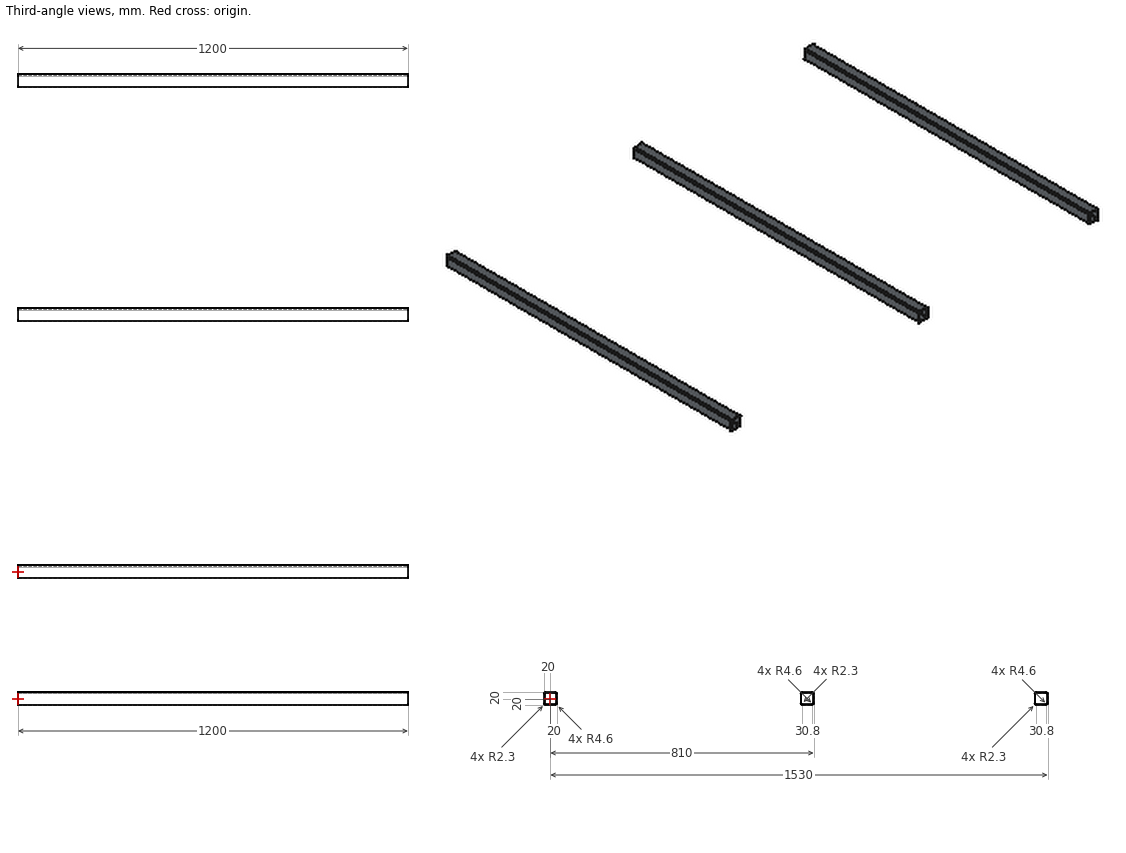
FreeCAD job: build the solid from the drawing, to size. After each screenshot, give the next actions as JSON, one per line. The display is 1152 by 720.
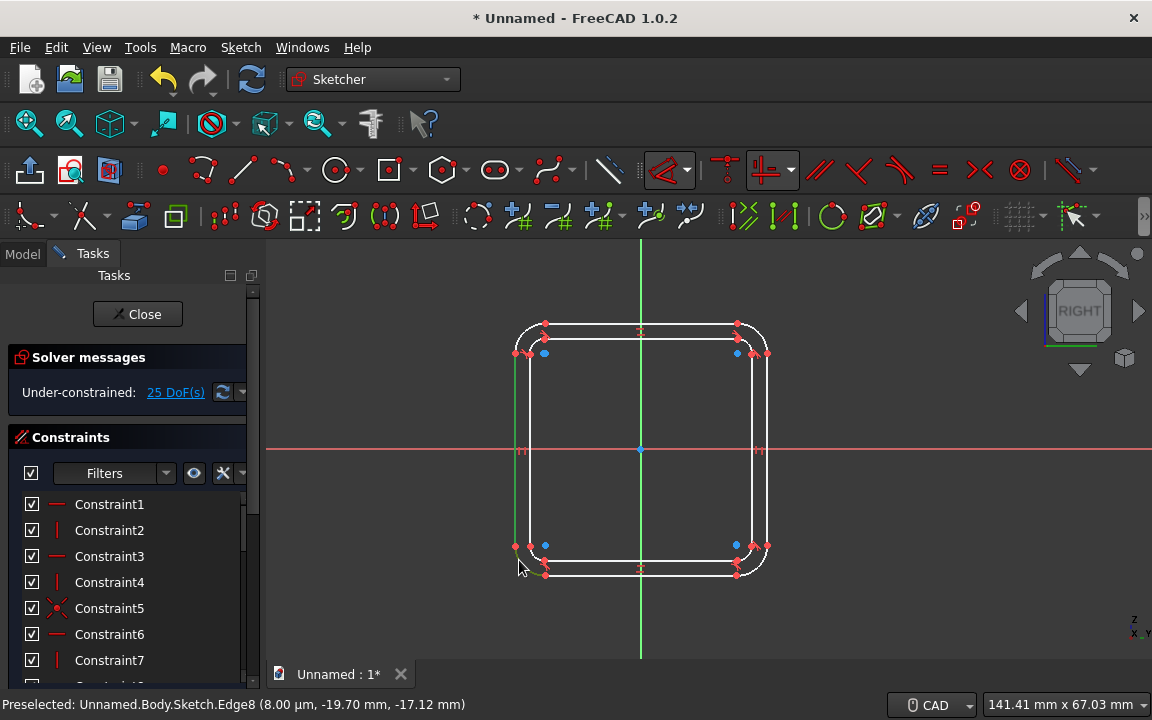
{"action": "key", "text": "t"}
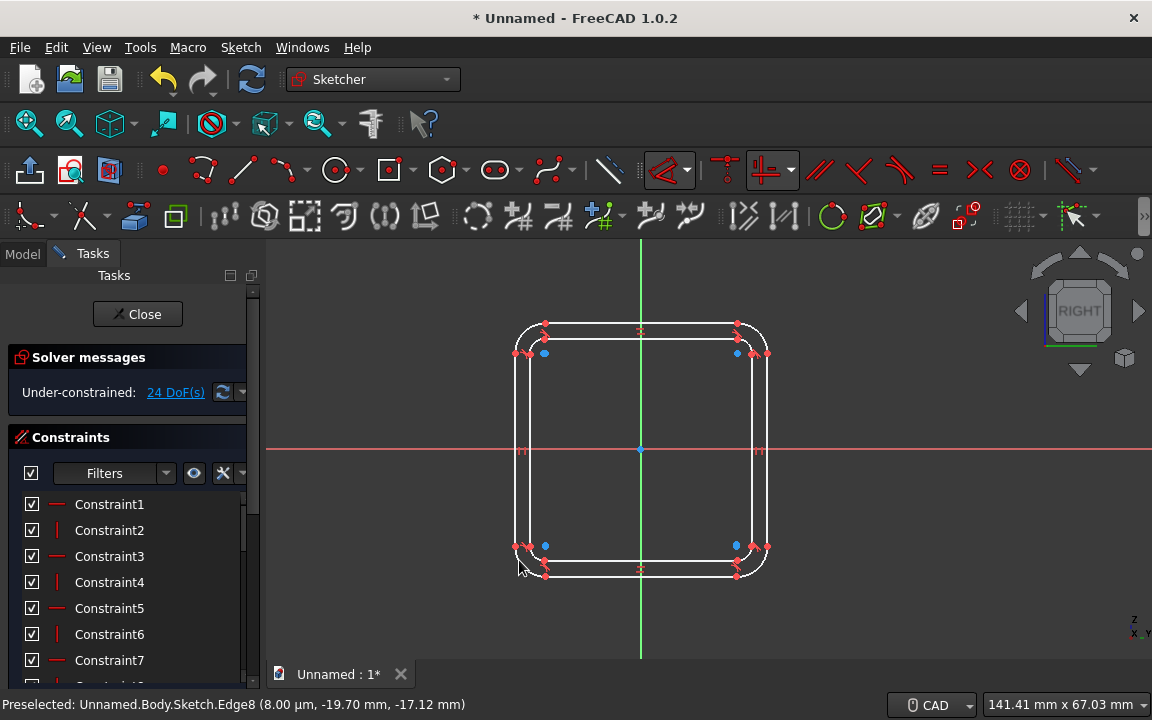
{"action": "left_click", "coordinate": [679, 561]}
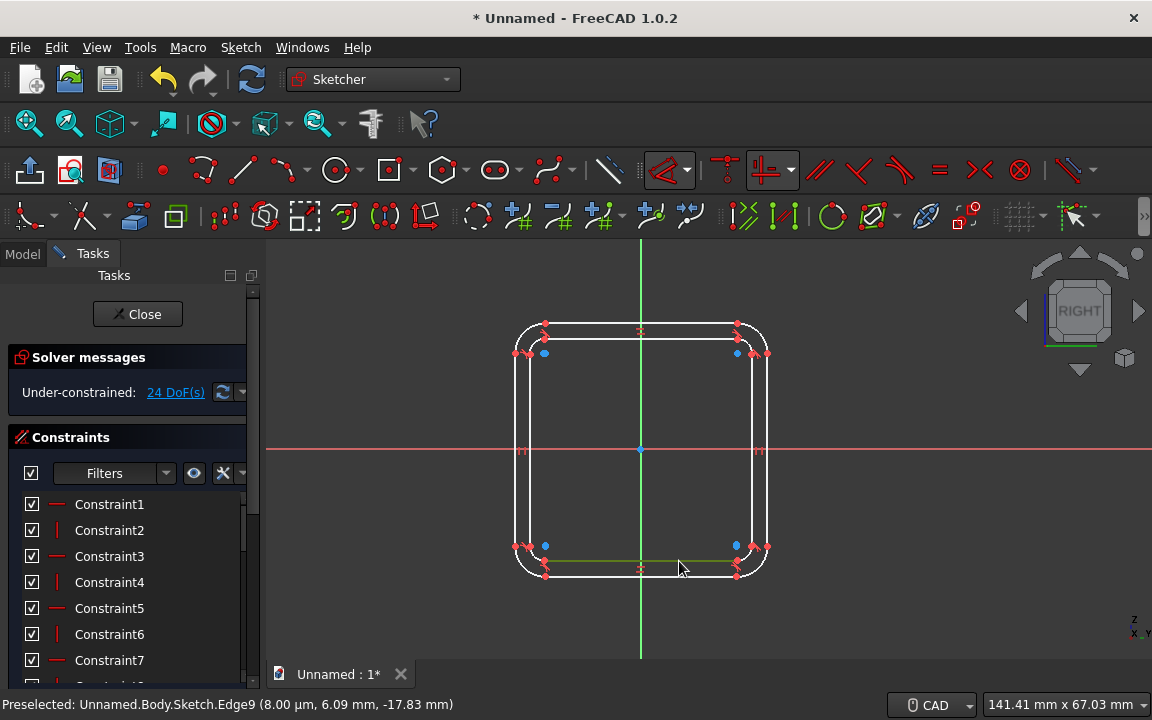
{"action": "scroll", "coordinate": [534, 557], "scroll_direction": "up", "scroll_amount": 2}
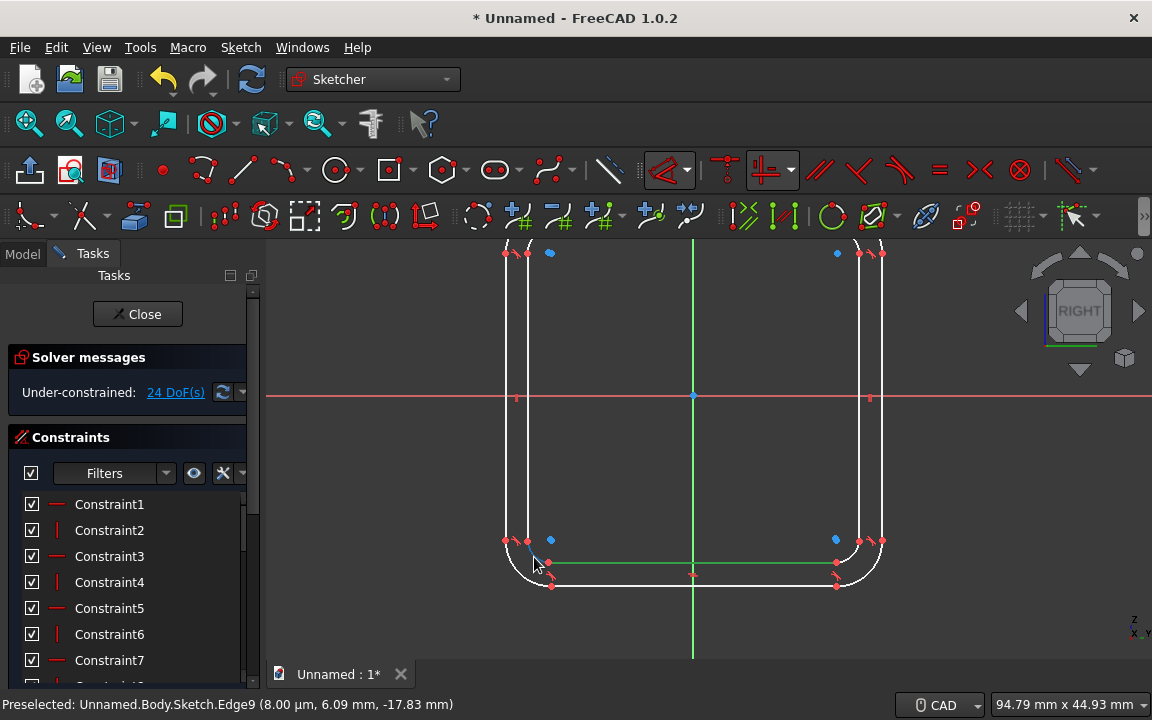
{"action": "left_click", "coordinate": [535, 556]}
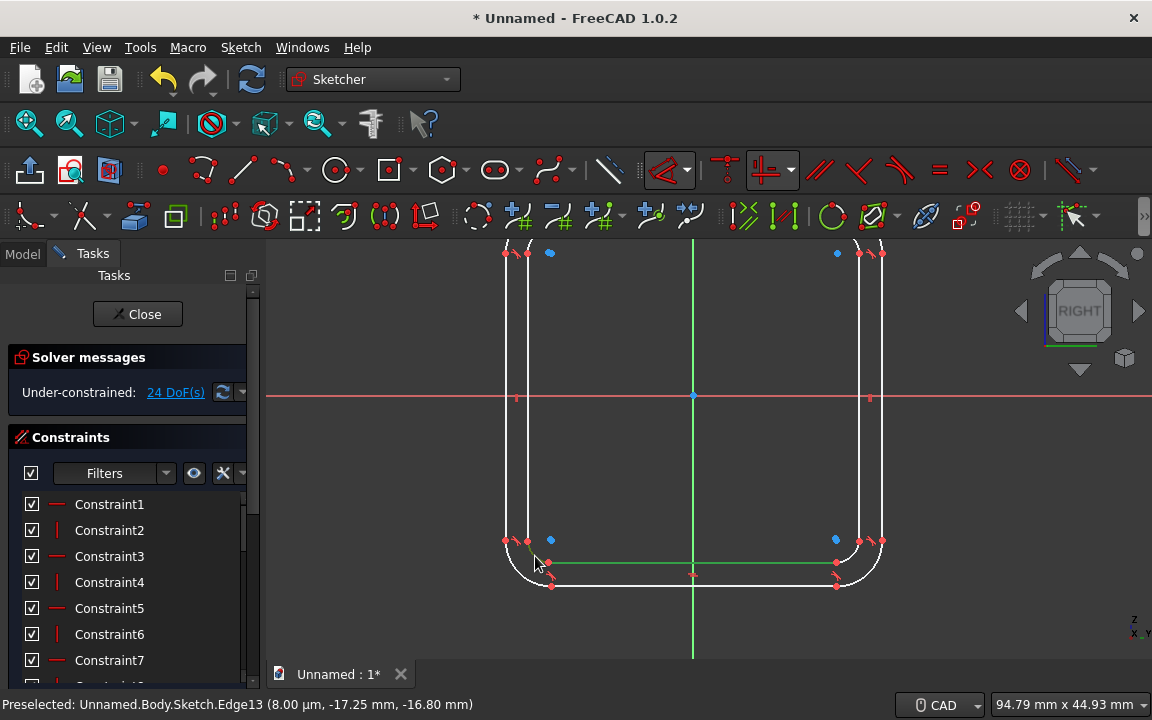
{"action": "key", "text": "t"}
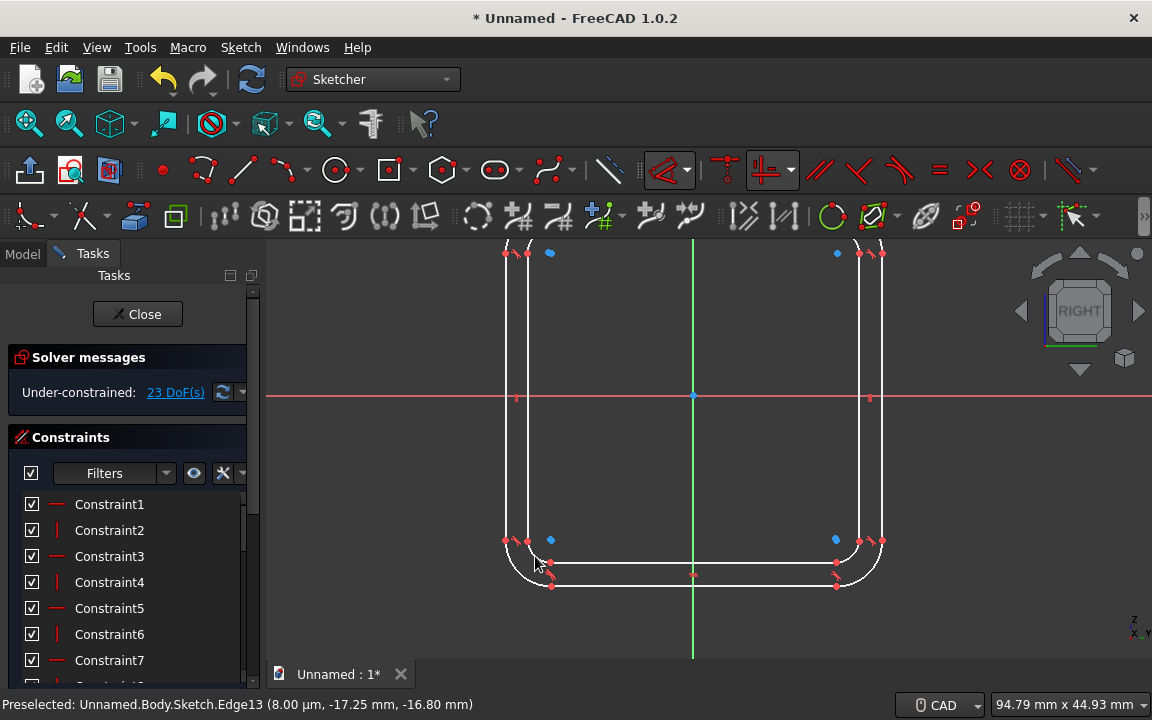
{"action": "left_click", "coordinate": [751, 563]}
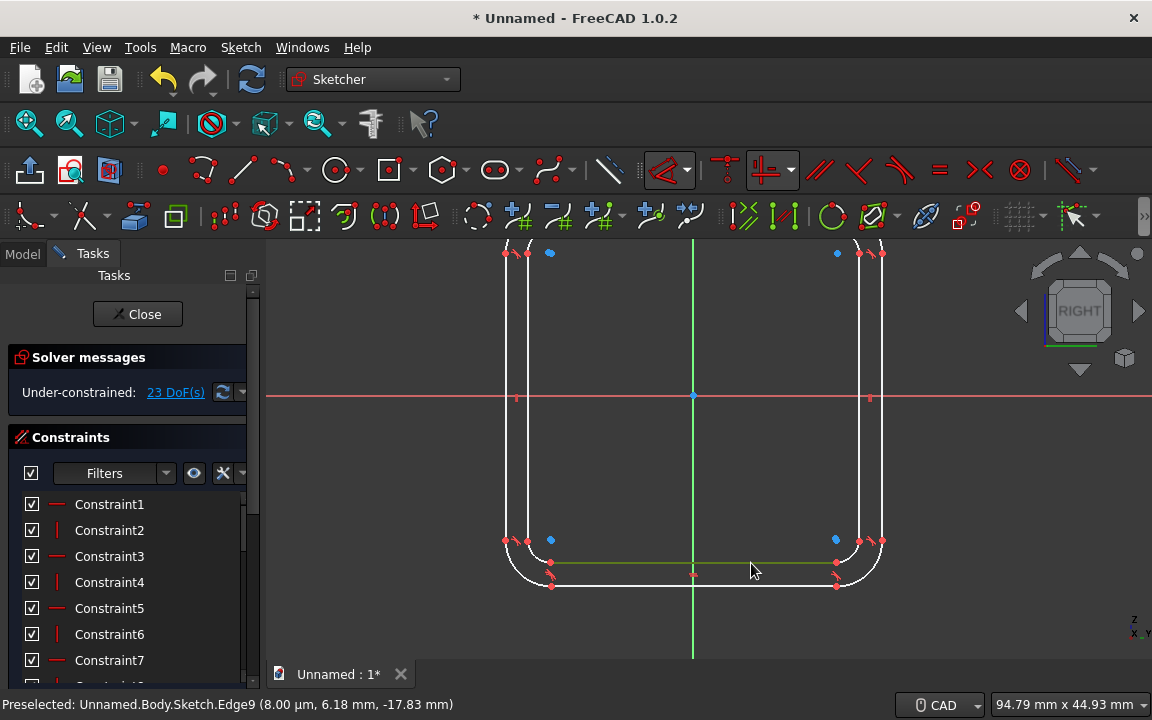
{"action": "scroll", "coordinate": [846, 560], "scroll_direction": "up", "scroll_amount": 2}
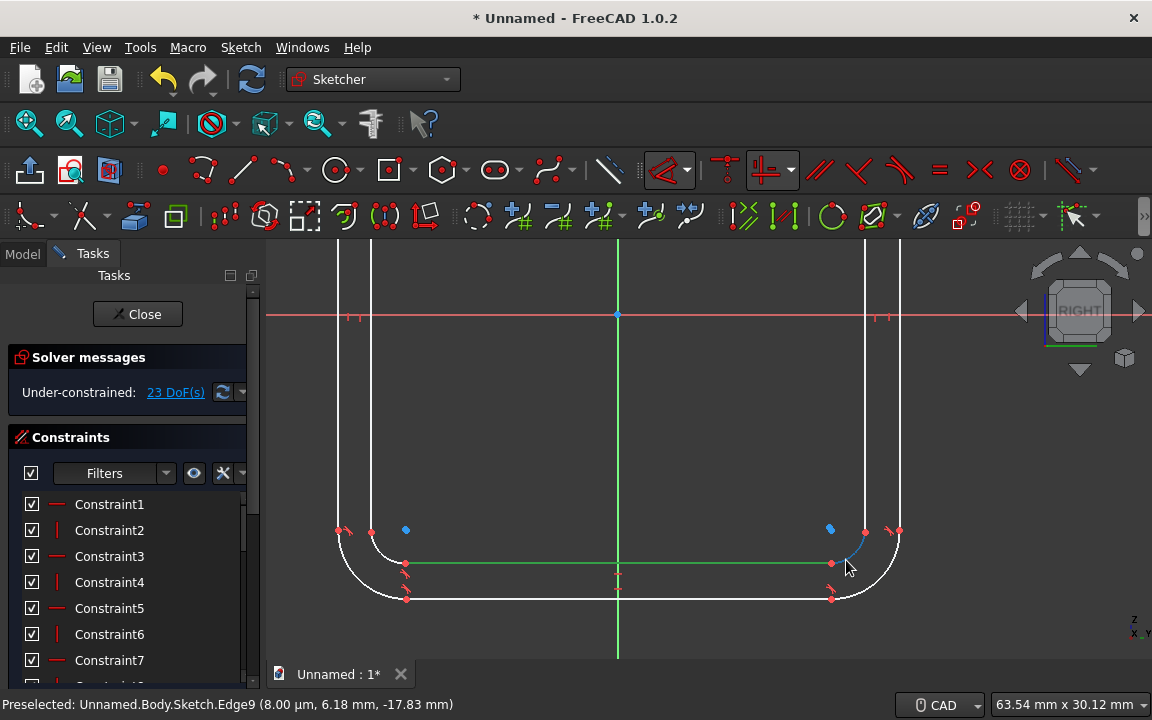
{"action": "left_click", "coordinate": [846, 560]}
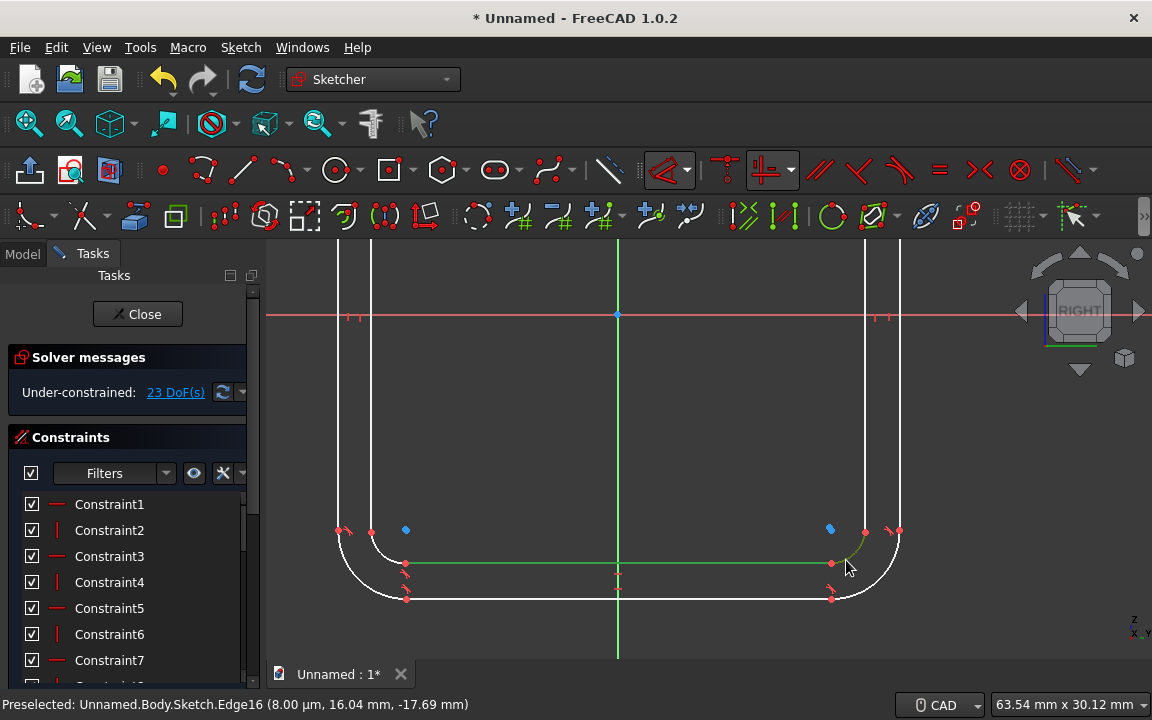
{"action": "key", "text": "t"}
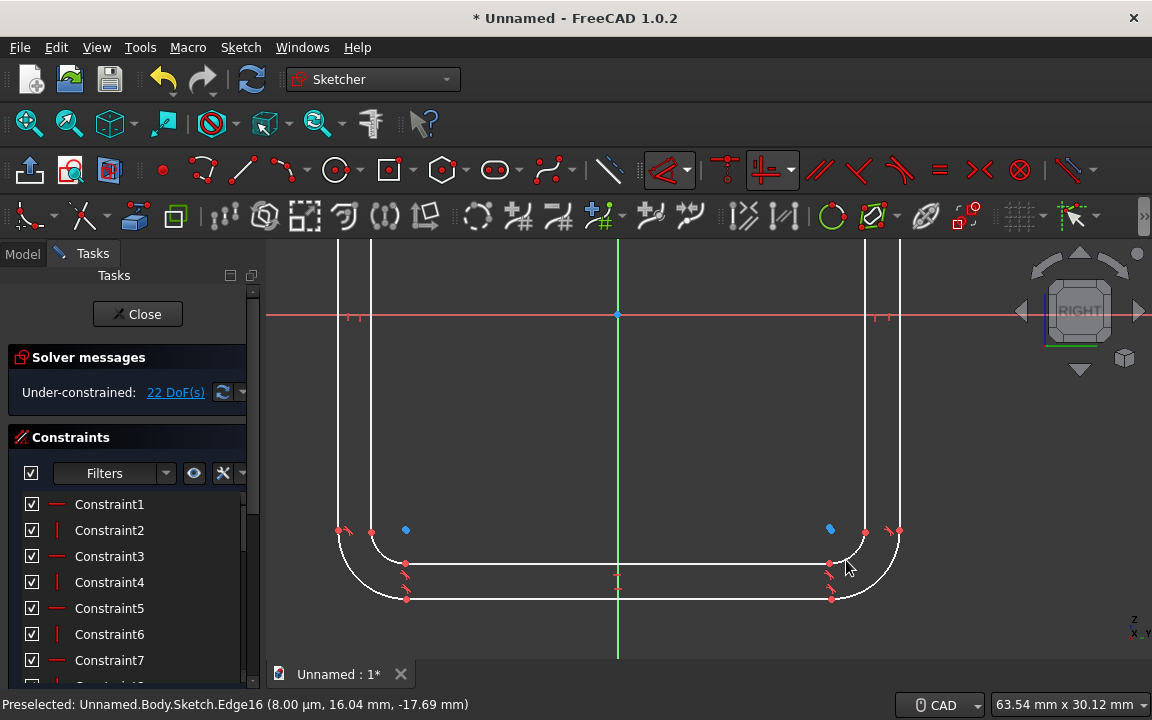
{"action": "left_click", "coordinate": [371, 403]}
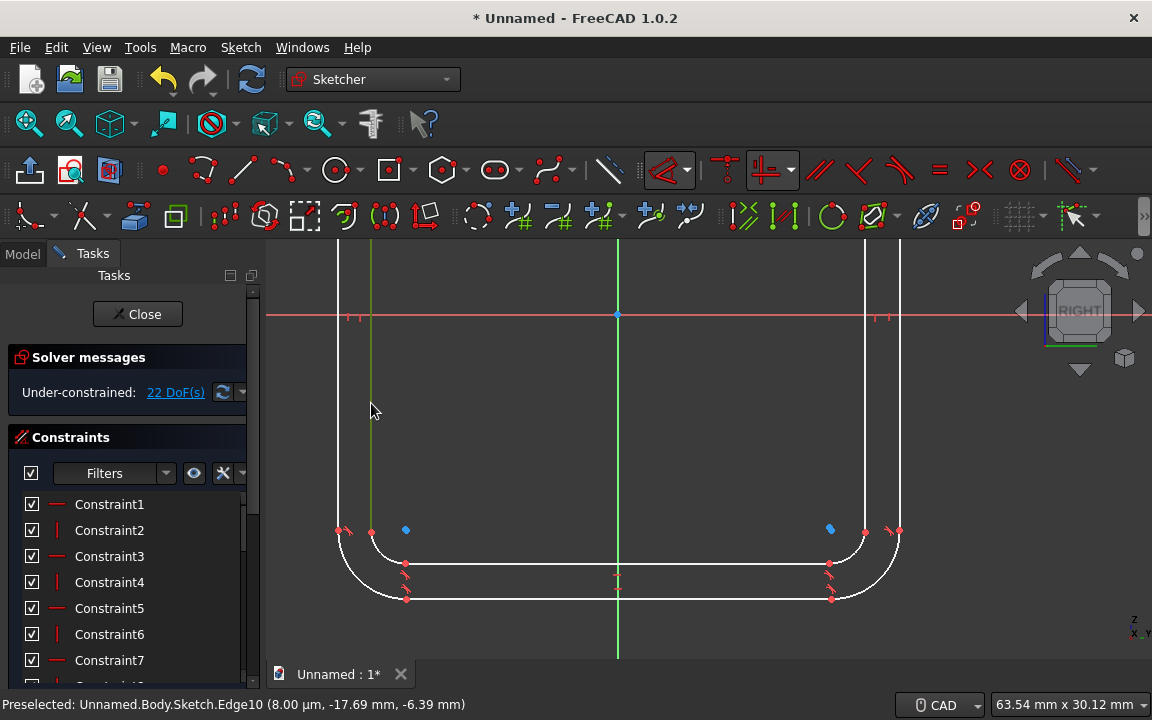
{"action": "left_click", "coordinate": [376, 547]}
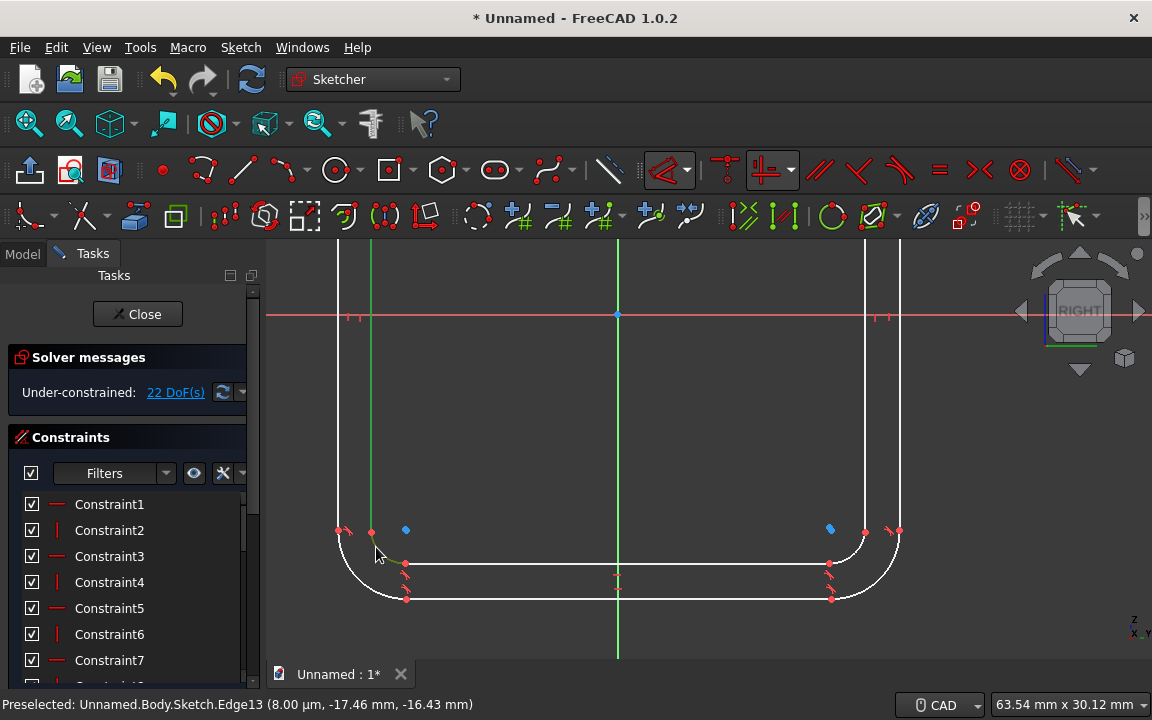
{"action": "key", "text": "t"}